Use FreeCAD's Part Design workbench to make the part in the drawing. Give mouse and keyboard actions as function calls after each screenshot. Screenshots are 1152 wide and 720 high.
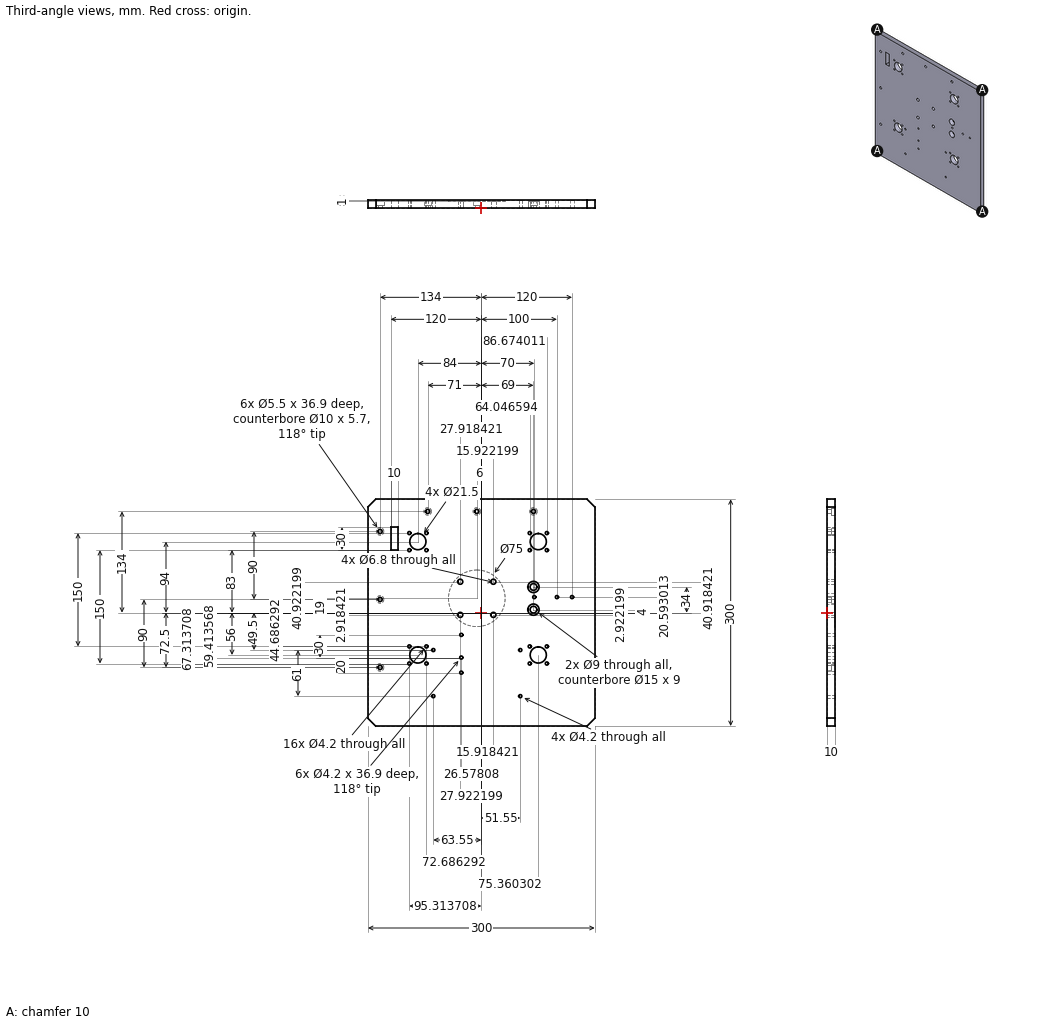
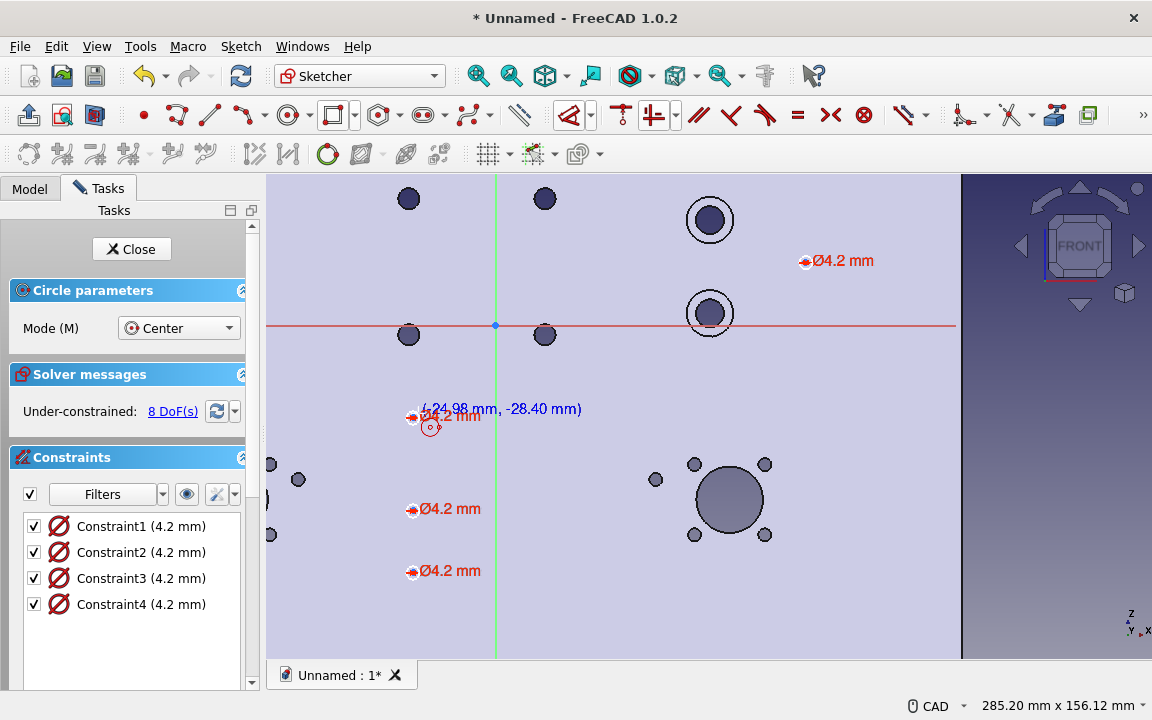
scroll(868, 262, up, 7)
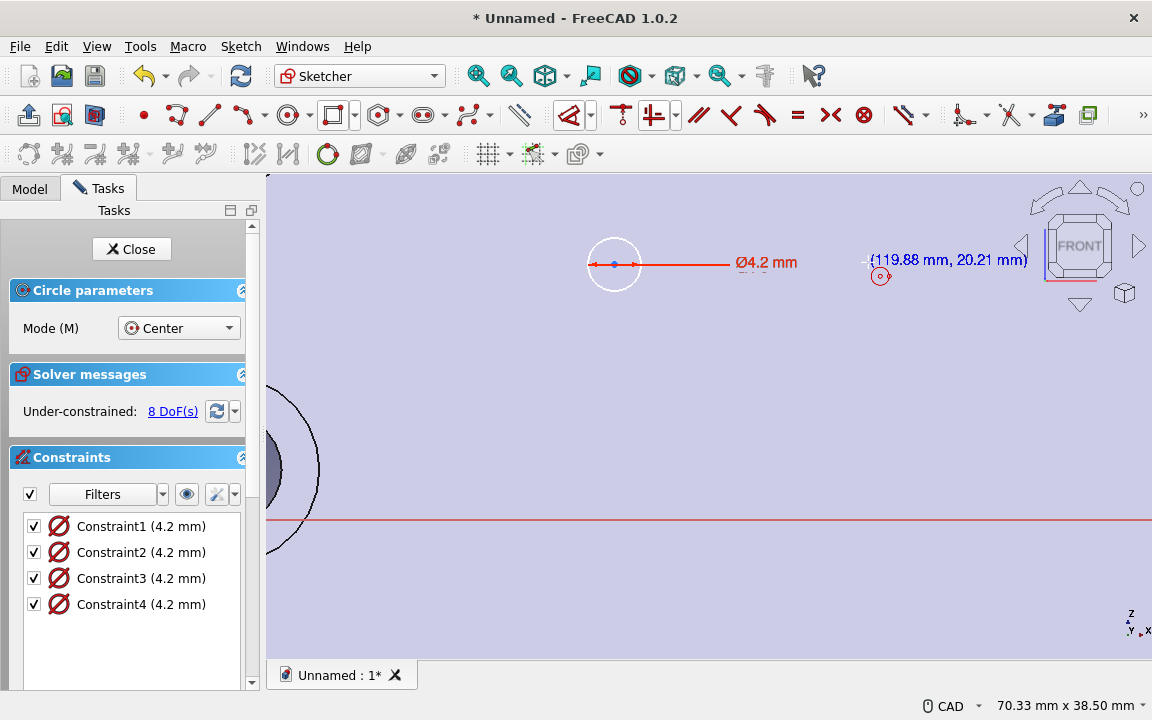
scroll(868, 261, down, 7)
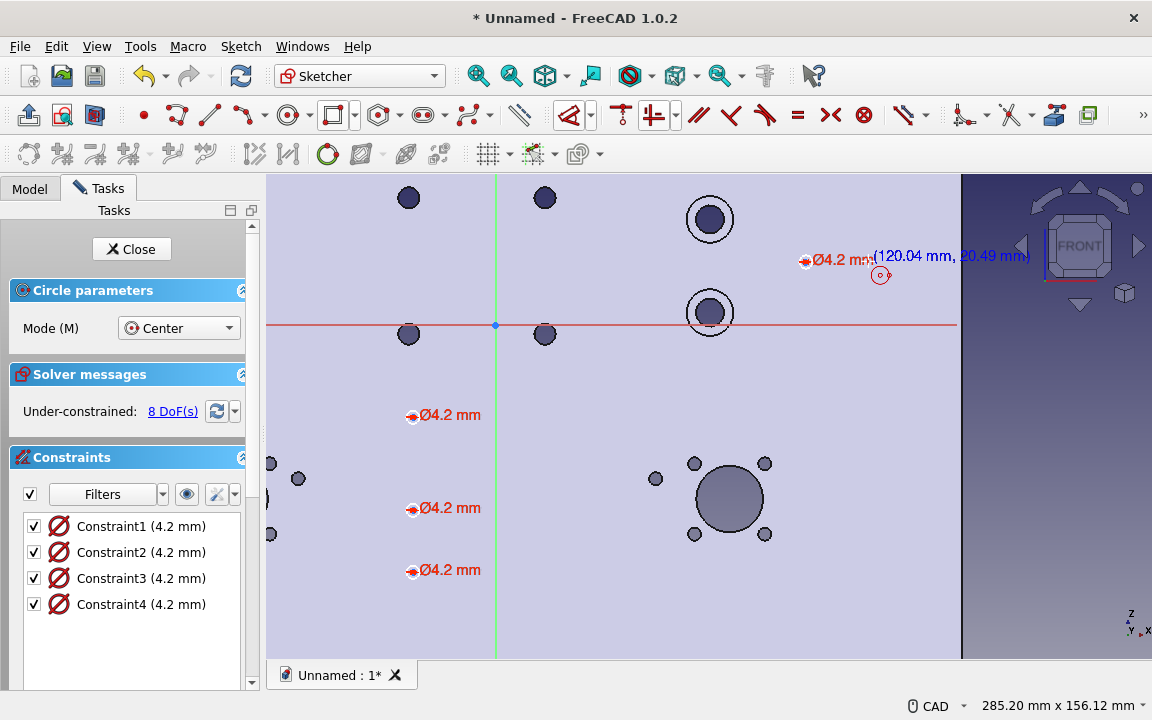
click(868, 261)
move(873, 256)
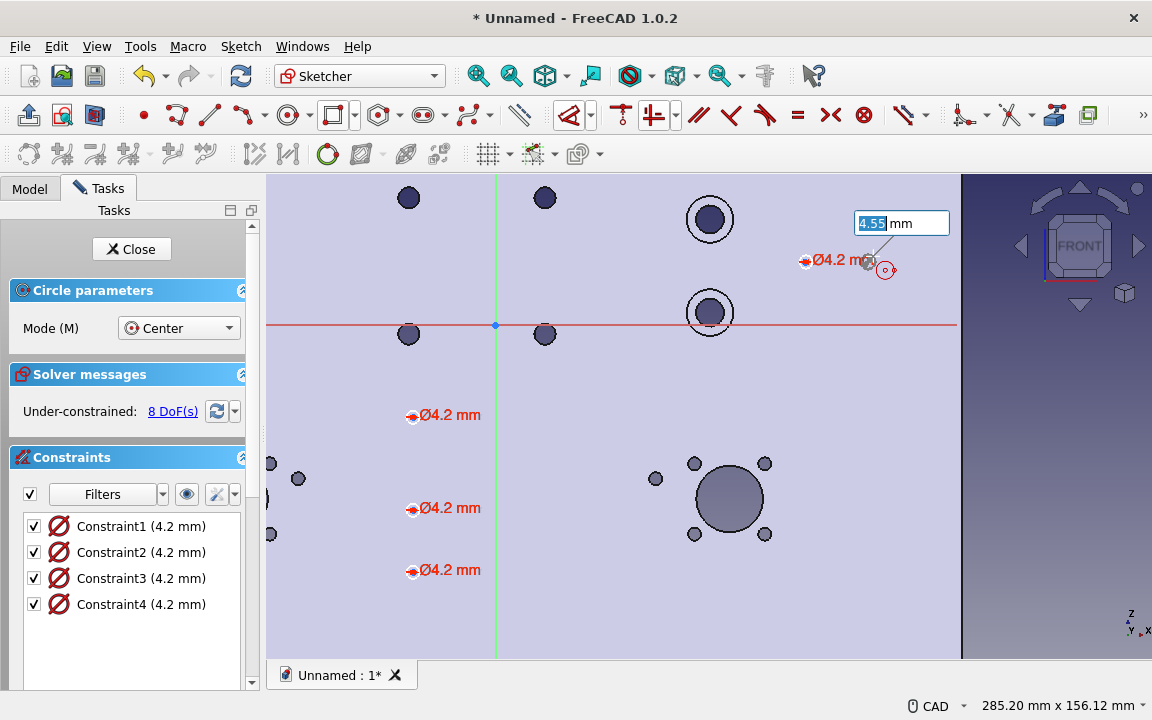
text(4.2)
key(Return)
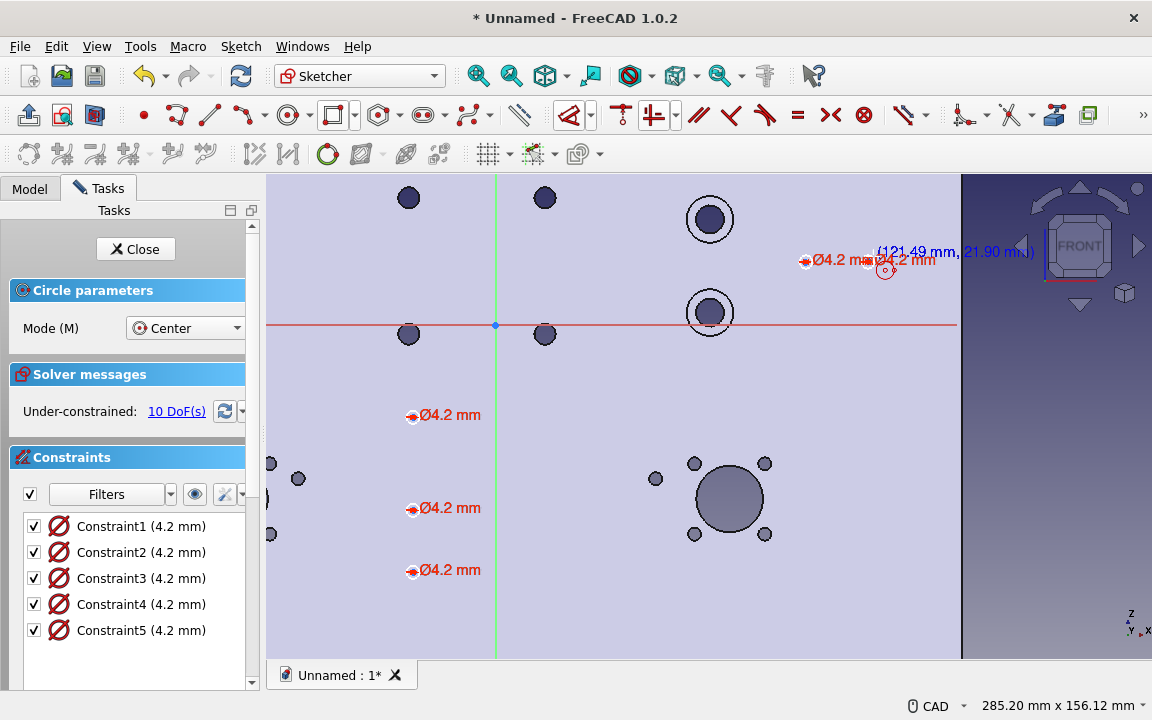
scroll(713, 261, up, 7)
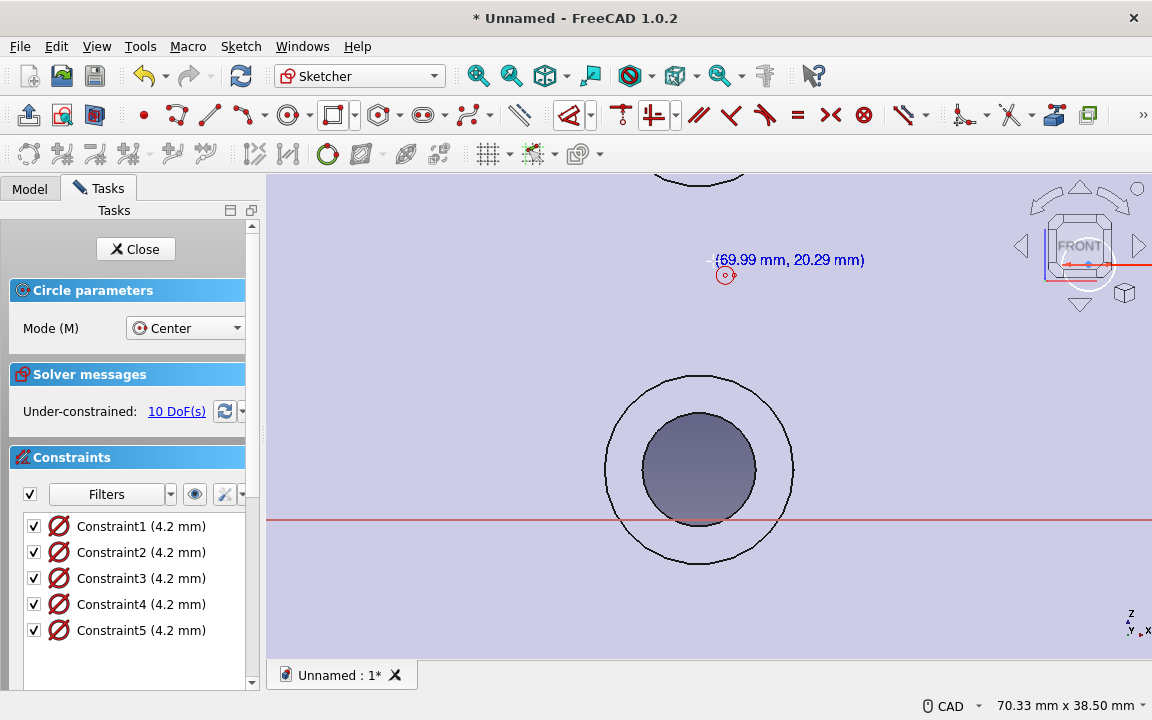
scroll(713, 261, down, 7)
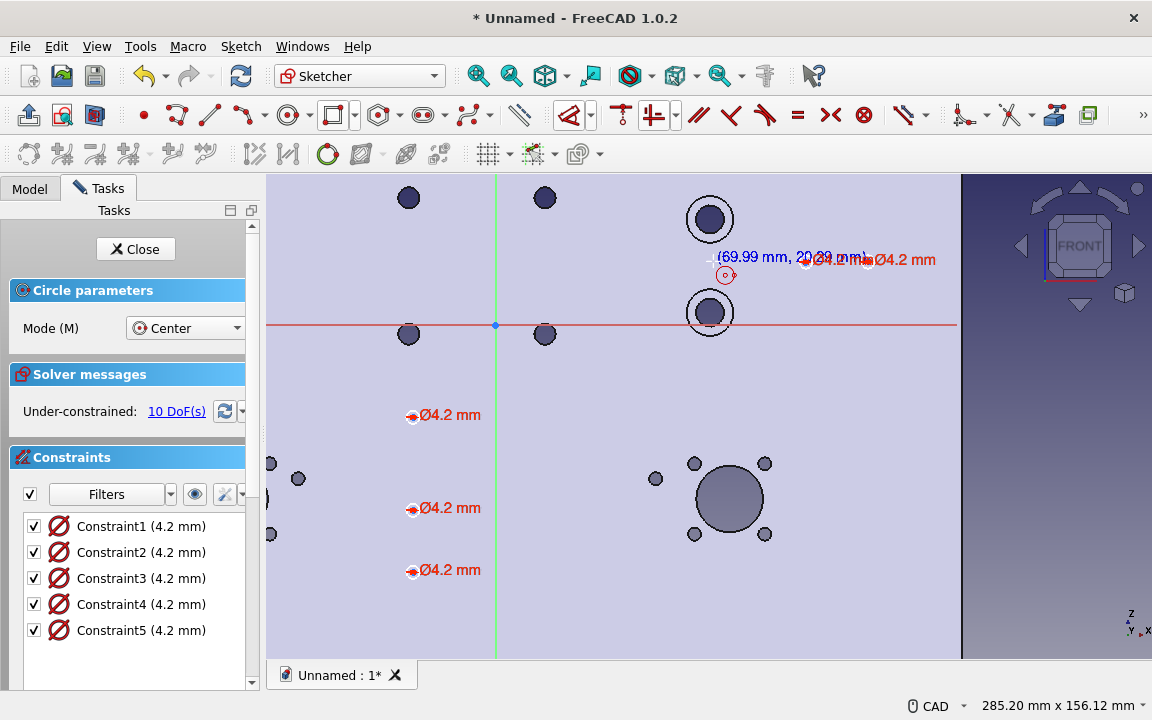
click(713, 261)
move(718, 256)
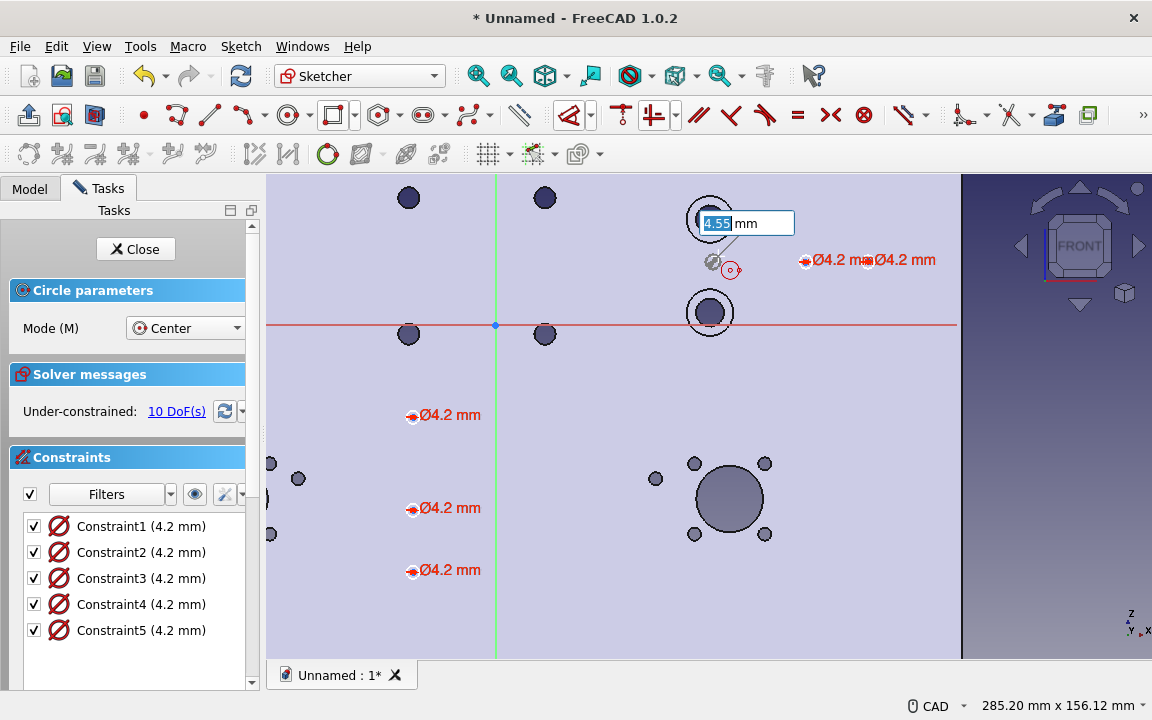
text(4.2)
key(Return)
key(Escape)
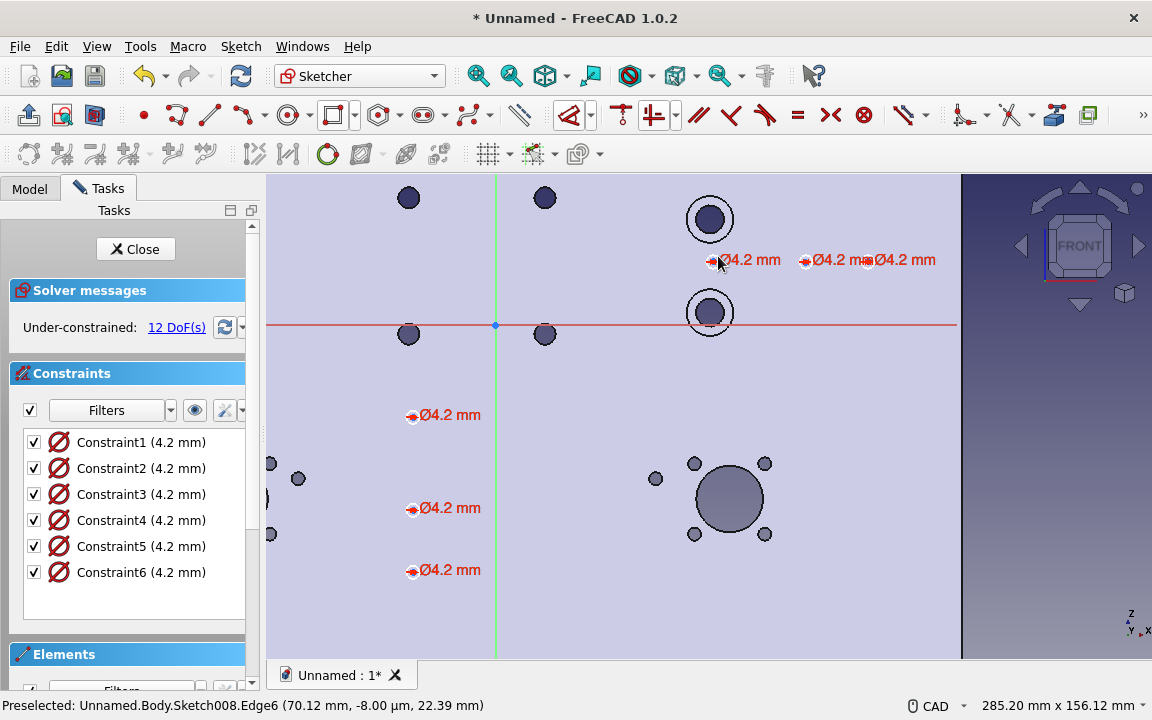
click(413, 510)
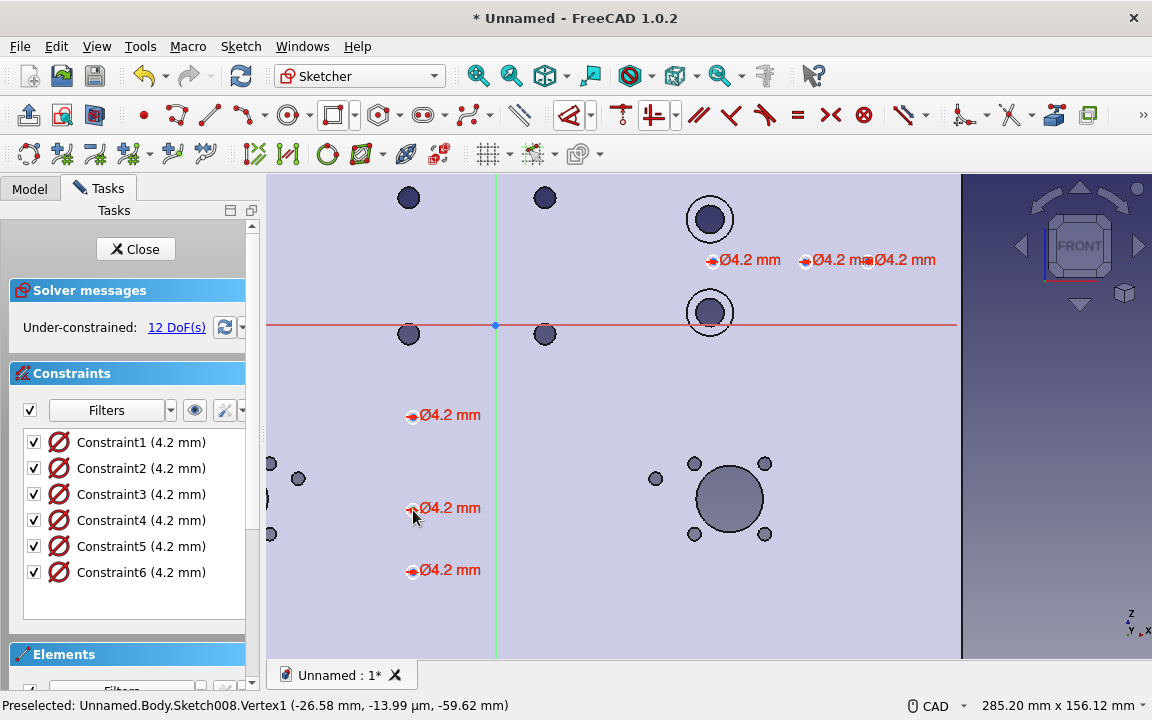
click(413, 572)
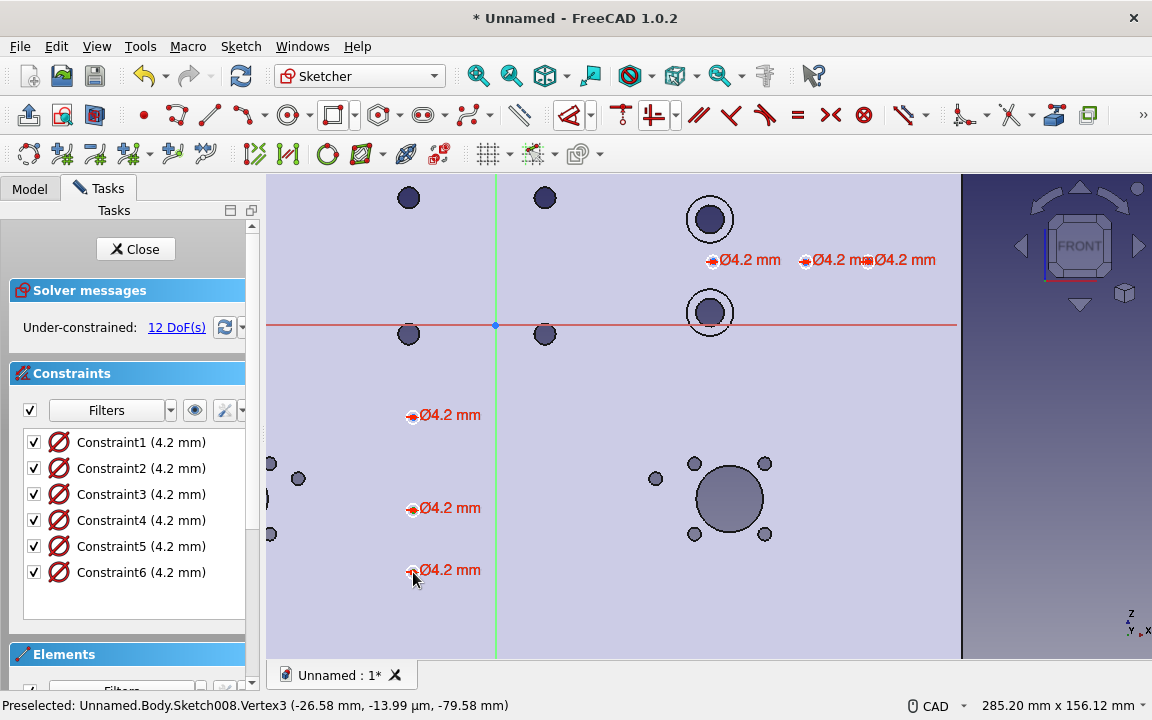
key(v)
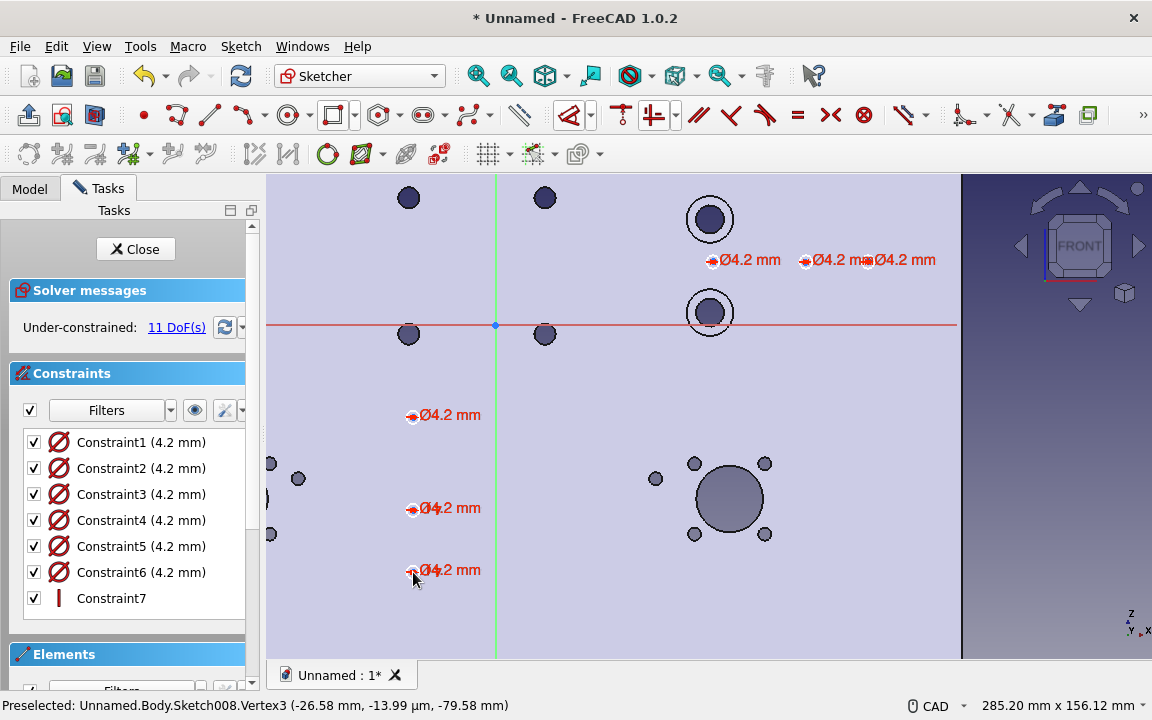
click(413, 510)